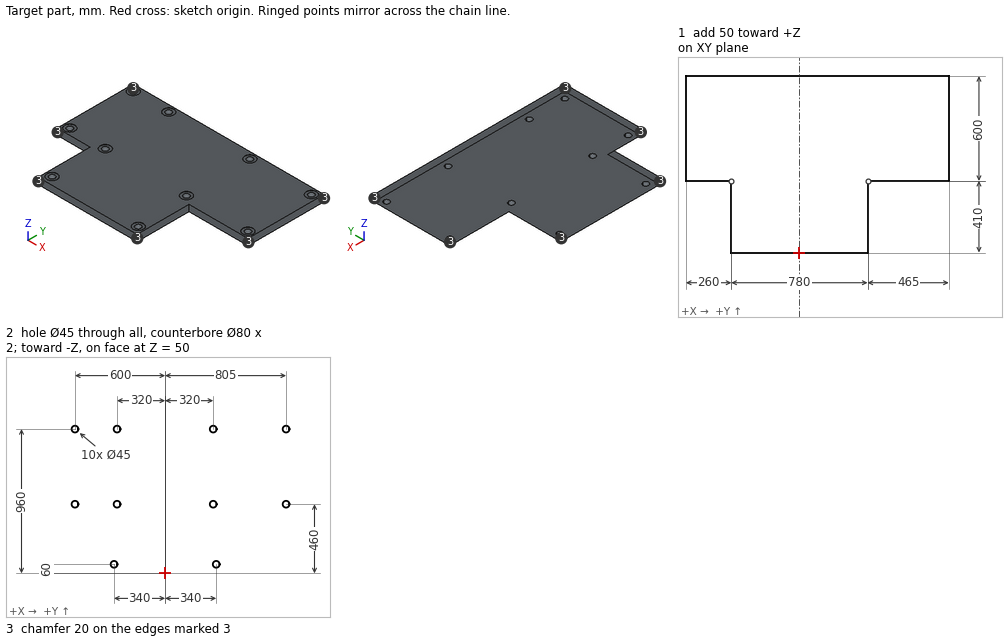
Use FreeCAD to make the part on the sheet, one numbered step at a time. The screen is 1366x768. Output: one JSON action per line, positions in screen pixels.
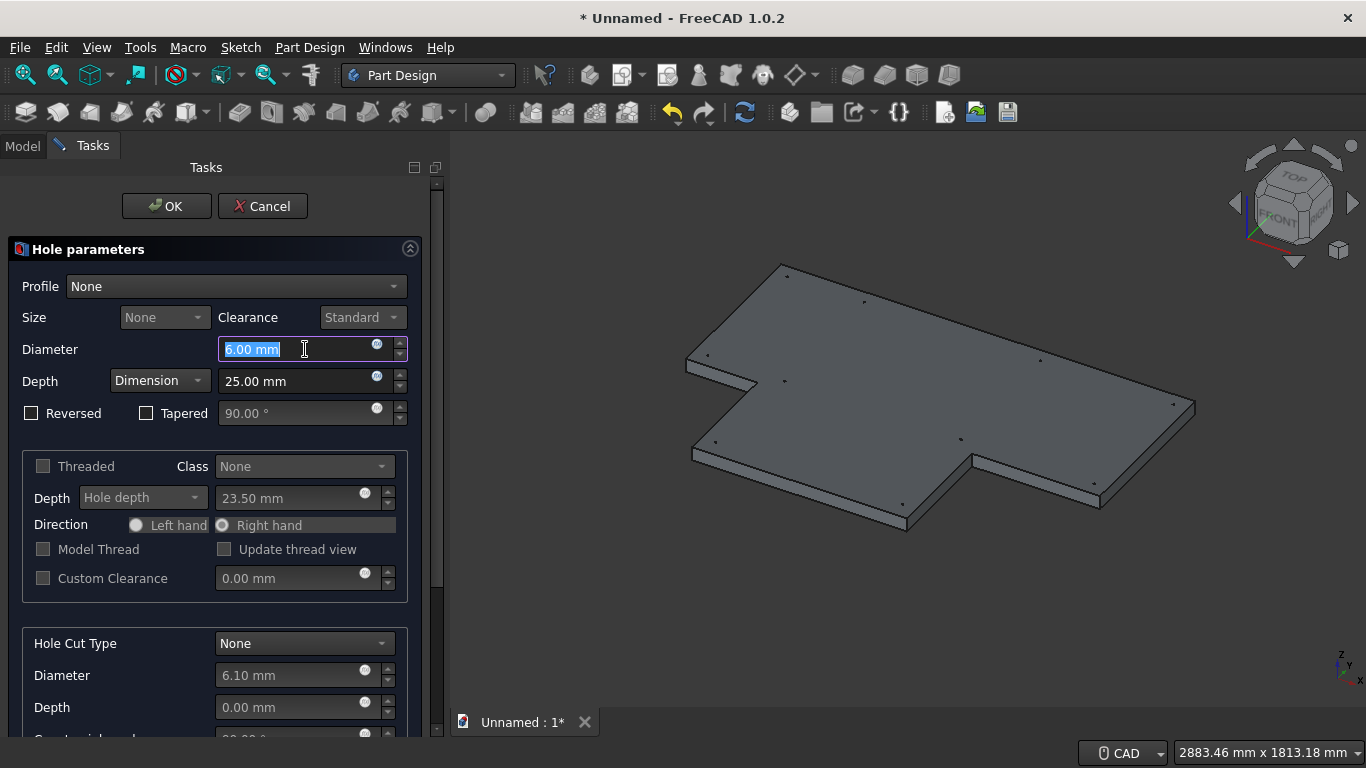
{"action": "type", "text": "45"}
{"action": "key", "text": "Tab"}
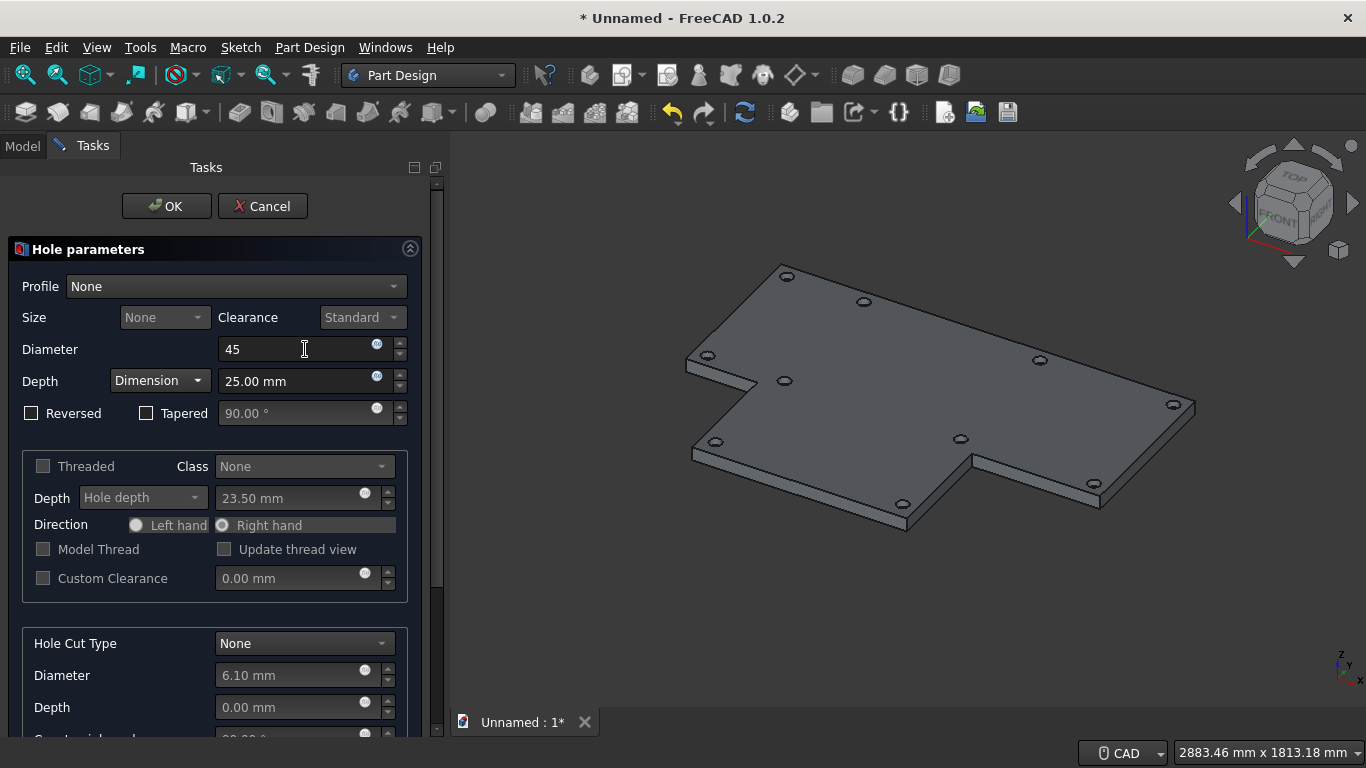
{"action": "left_click", "coordinate": [161, 380]}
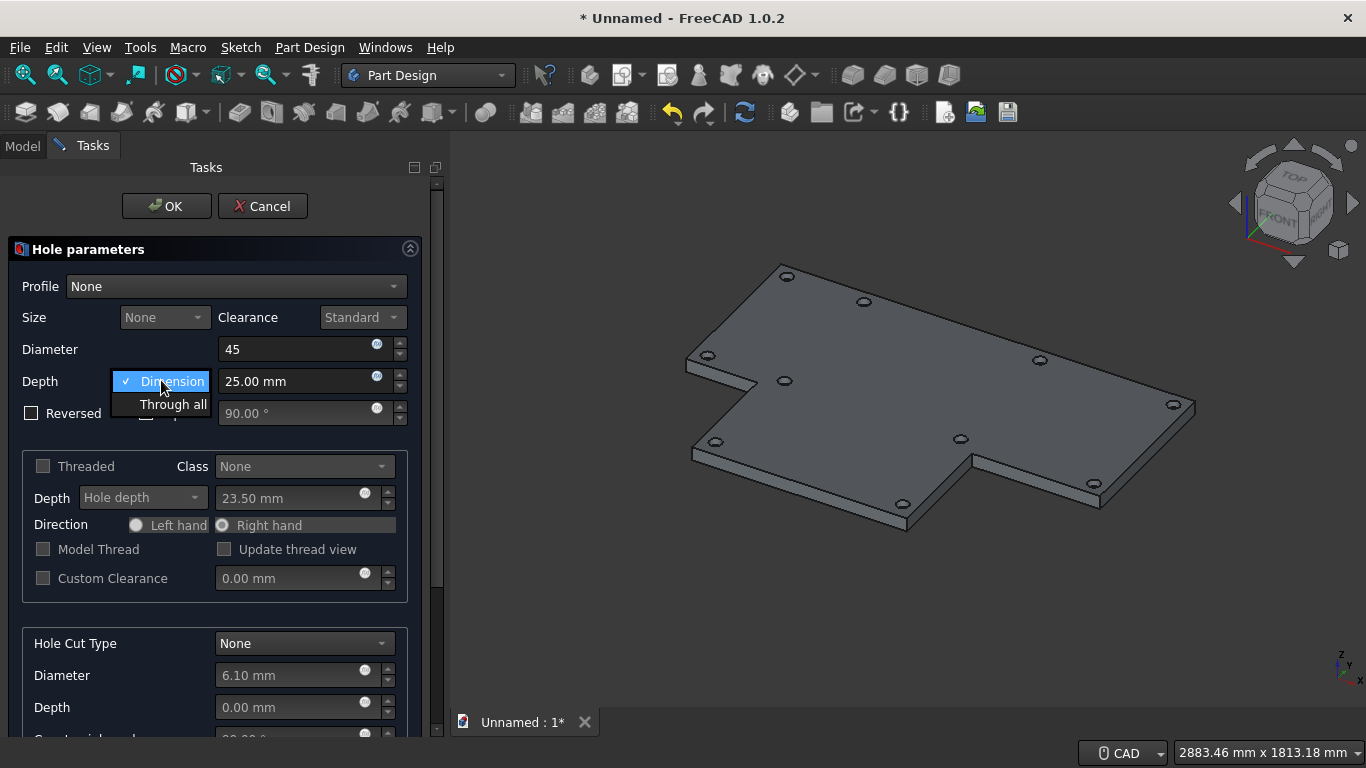
{"action": "left_click", "coordinate": [160, 404]}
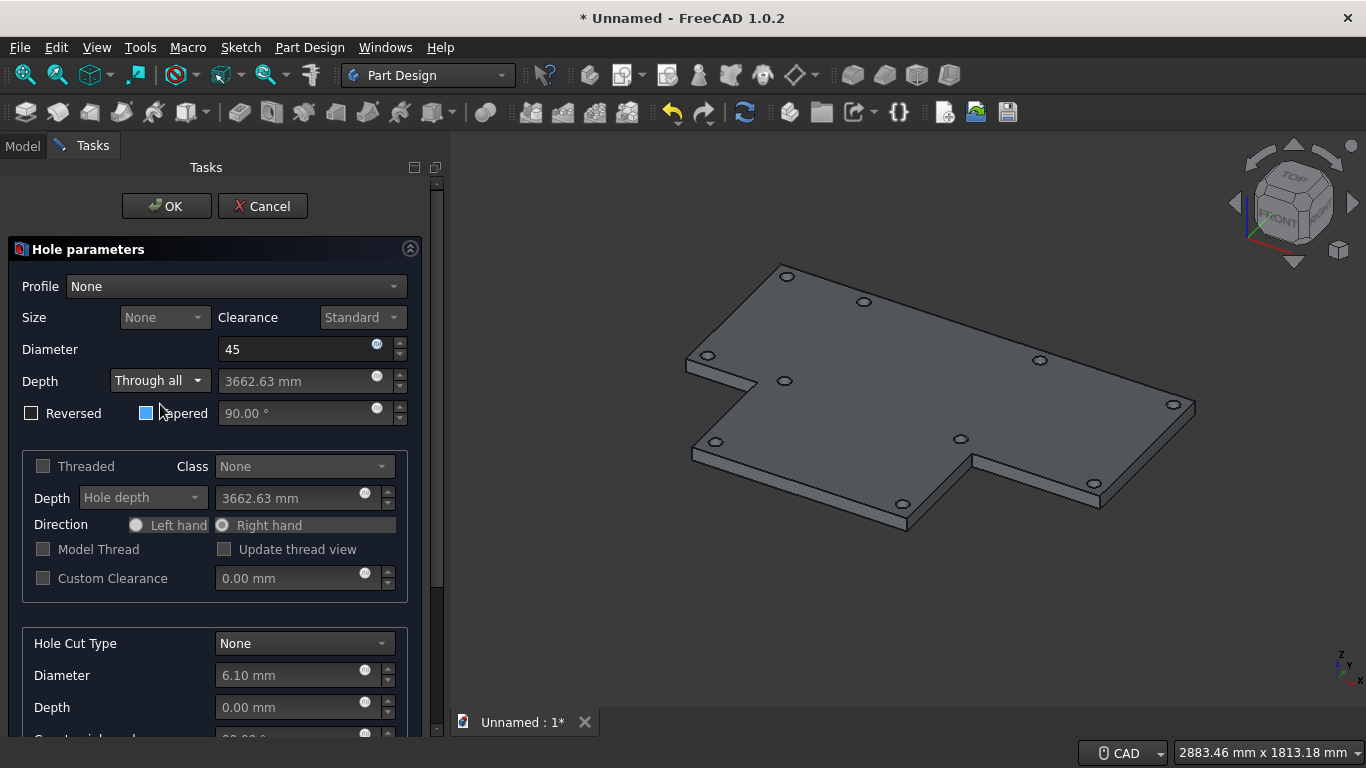
{"action": "left_click", "coordinate": [306, 644]}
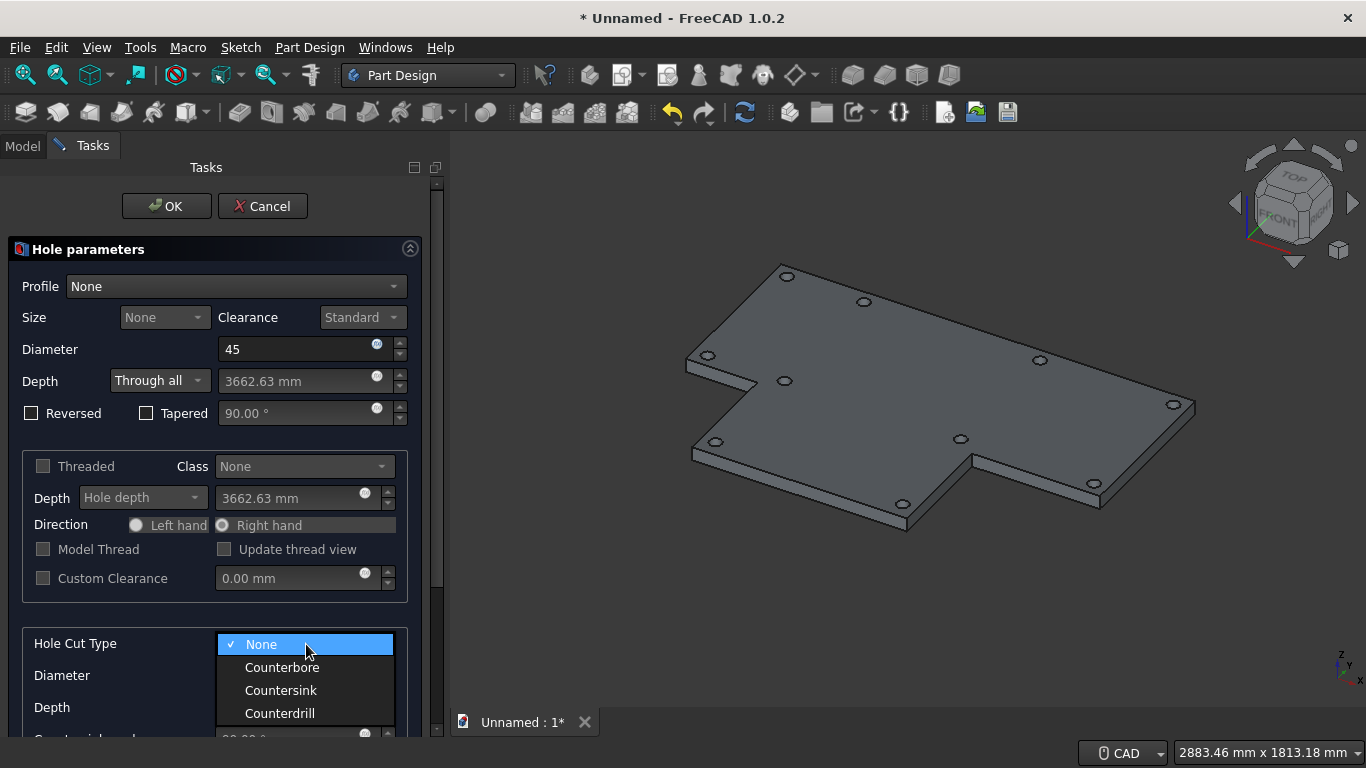
{"action": "left_click", "coordinate": [304, 668]}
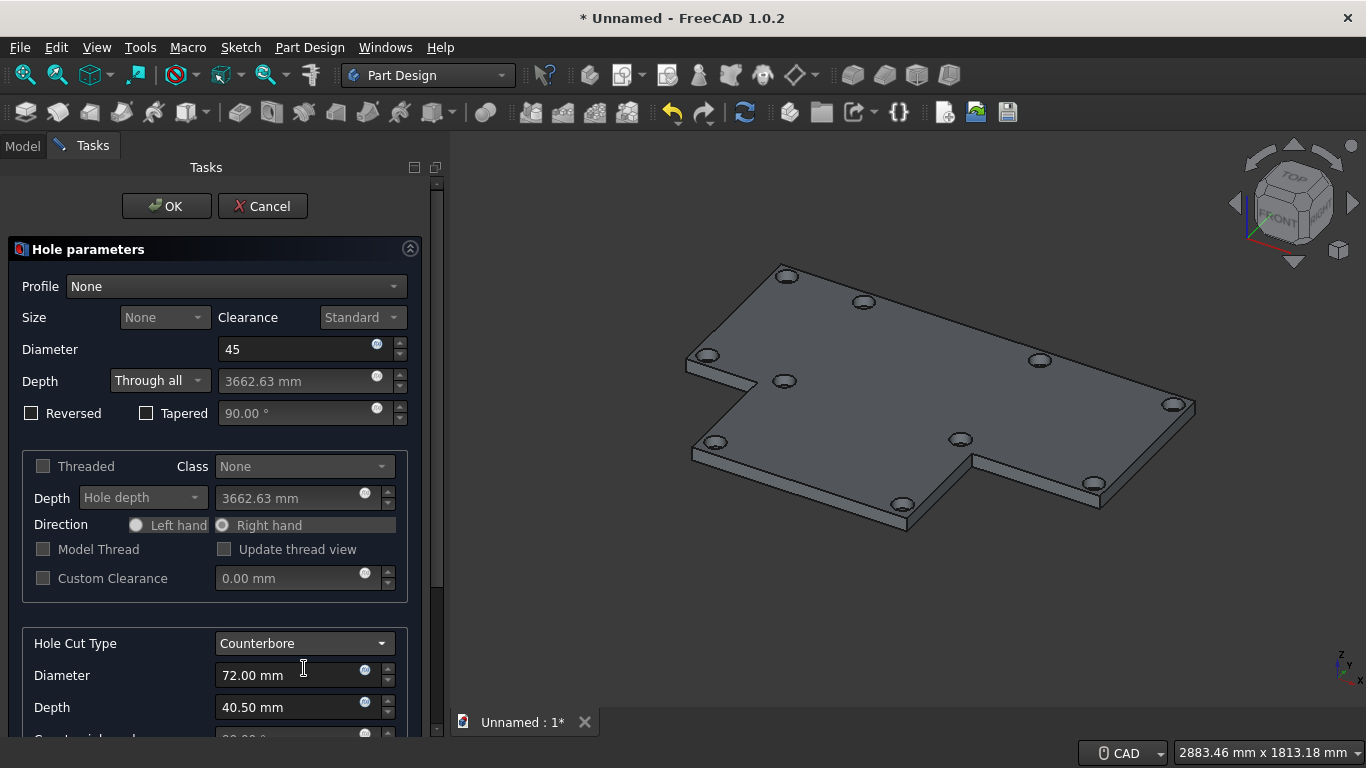
{"action": "triple_click", "coordinate": [298, 675]}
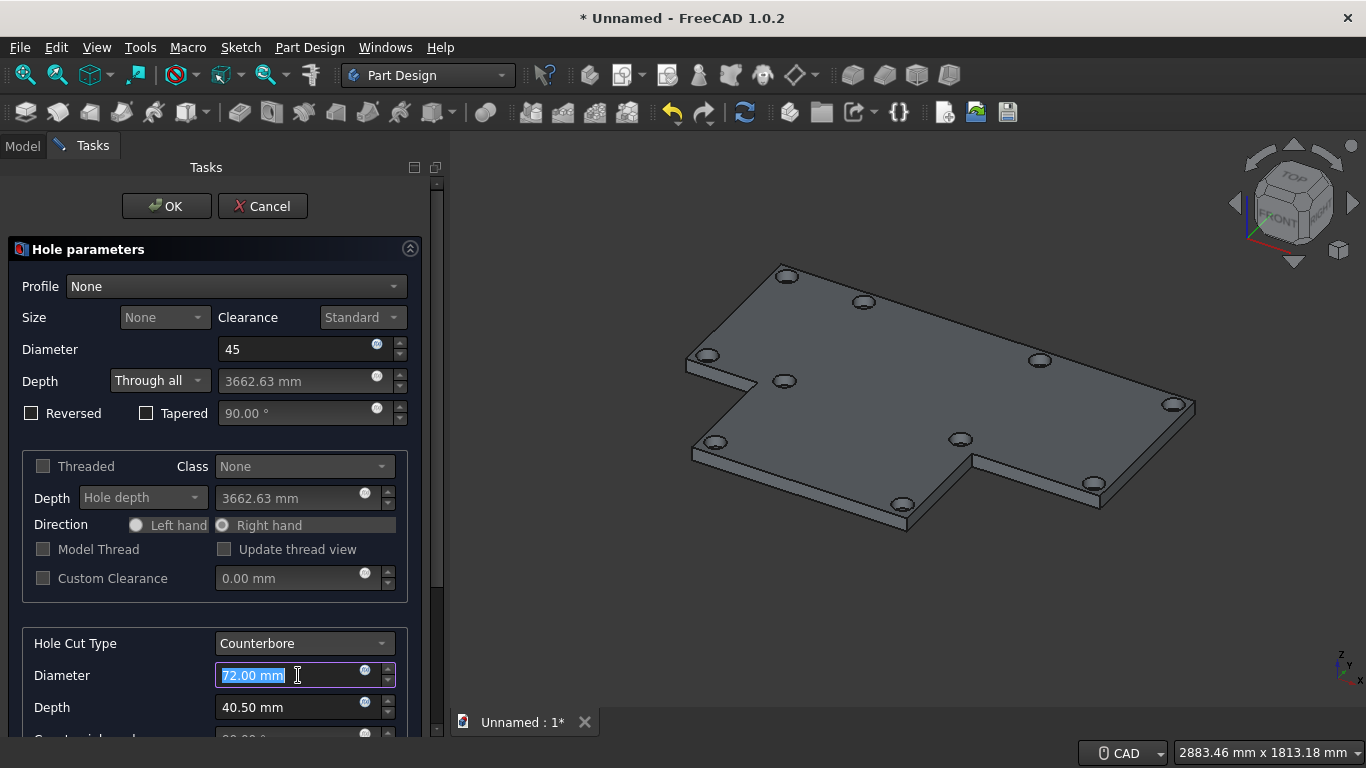
{"action": "type", "text": "80"}
{"action": "key", "text": "Tab"}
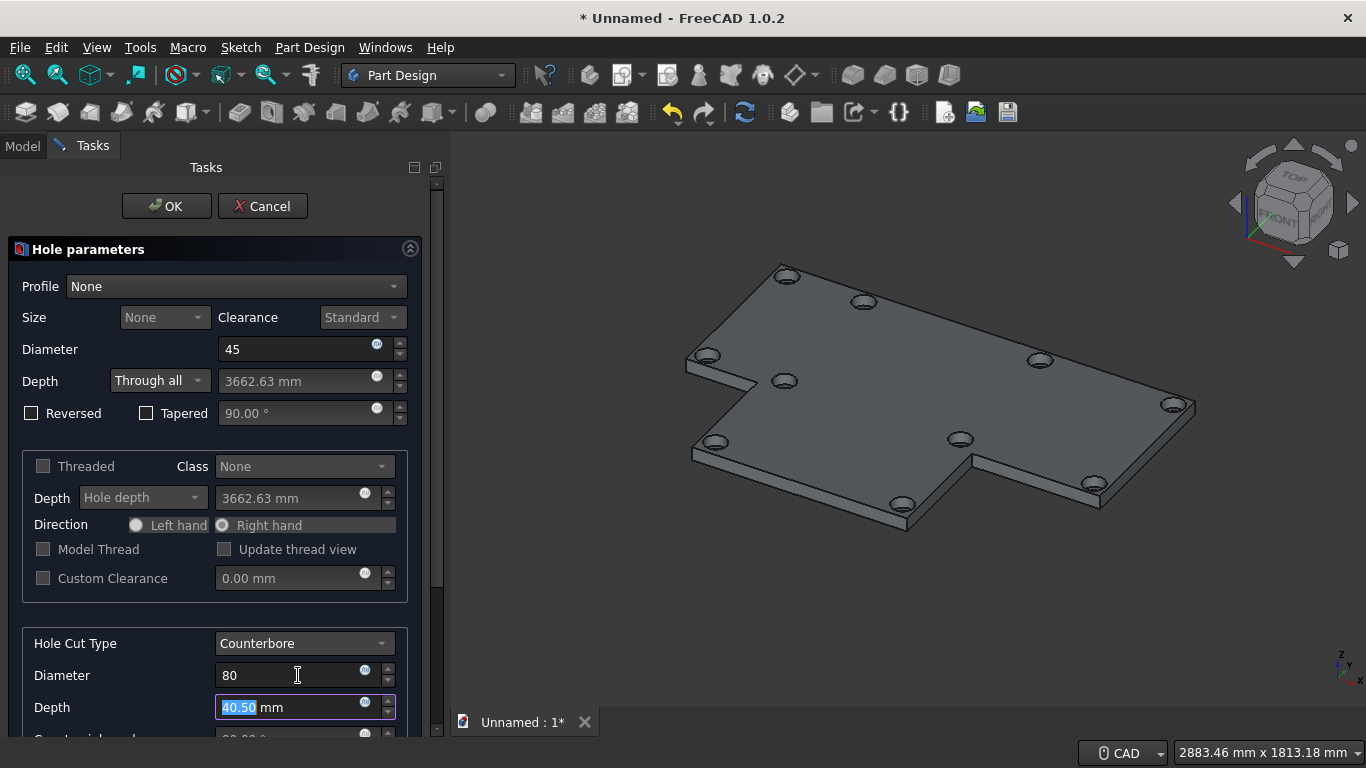
{"action": "type", "text": "2"}
{"action": "key", "text": "Tab"}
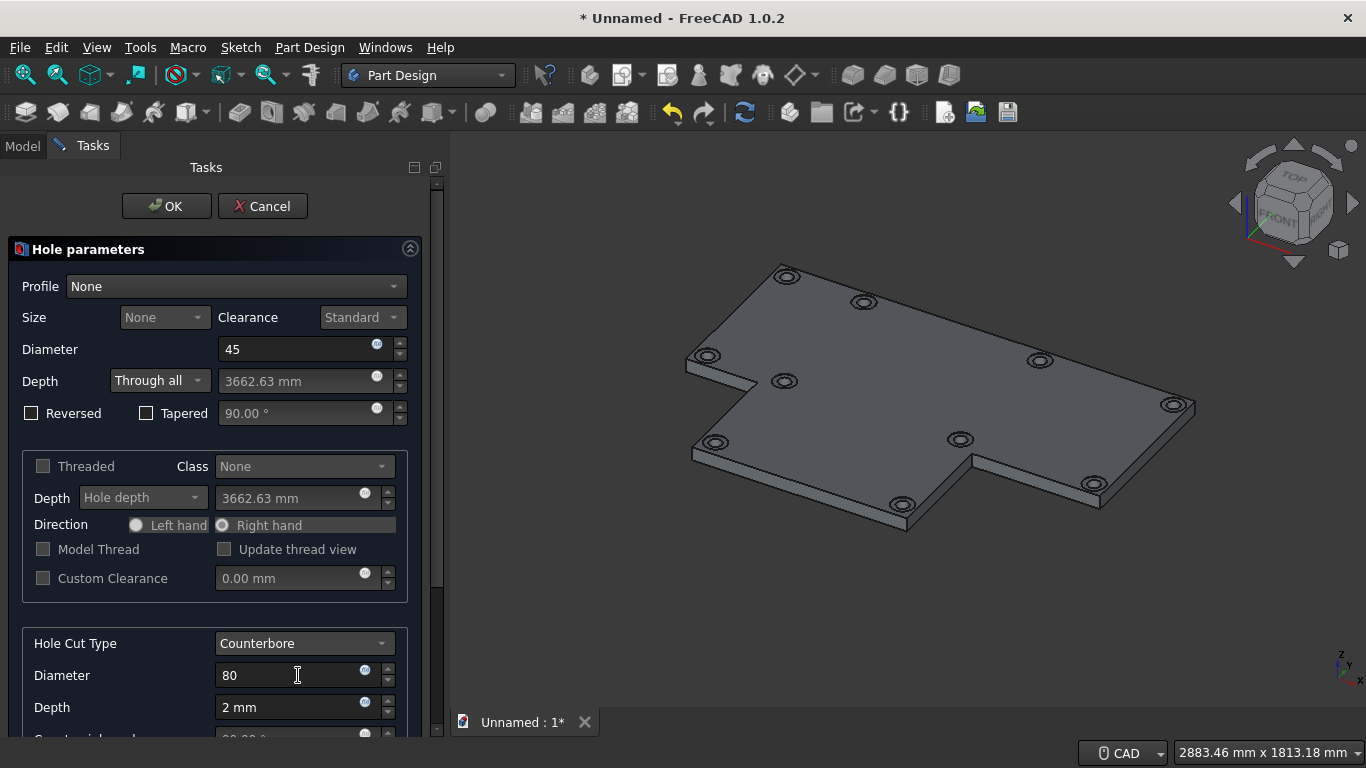
{"action": "left_click", "coordinate": [167, 206]}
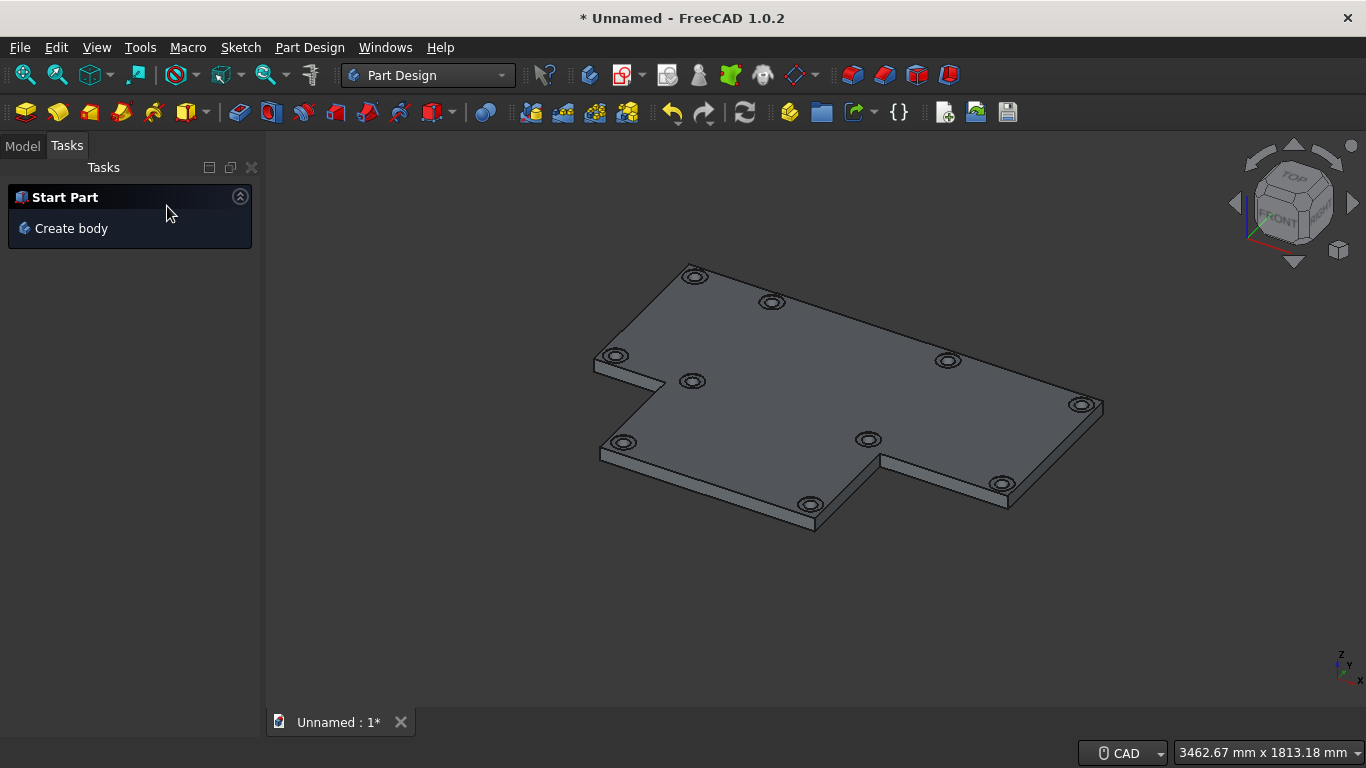
{"action": "left_click", "coordinate": [1008, 502]}